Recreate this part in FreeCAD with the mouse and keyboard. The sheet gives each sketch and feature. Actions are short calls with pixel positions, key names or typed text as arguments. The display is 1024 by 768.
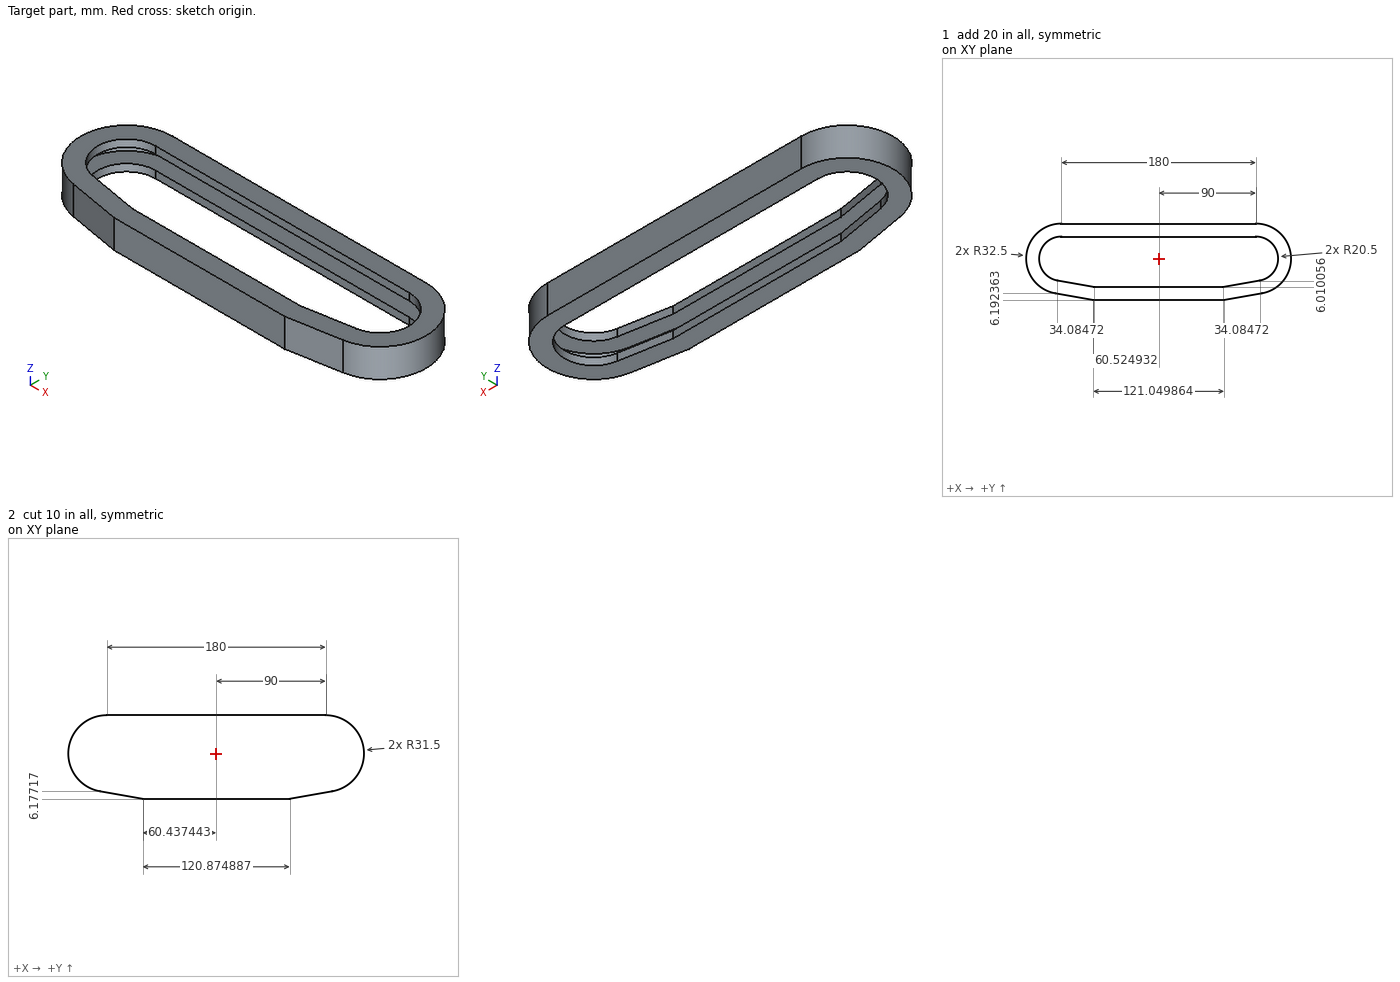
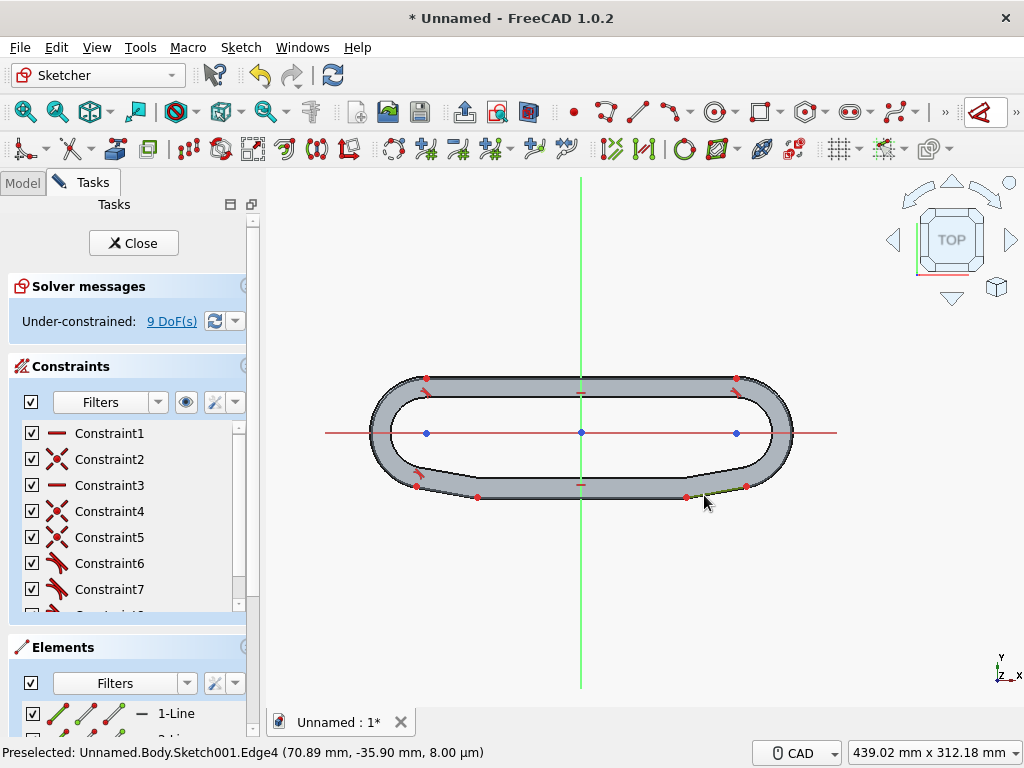
click(784, 460)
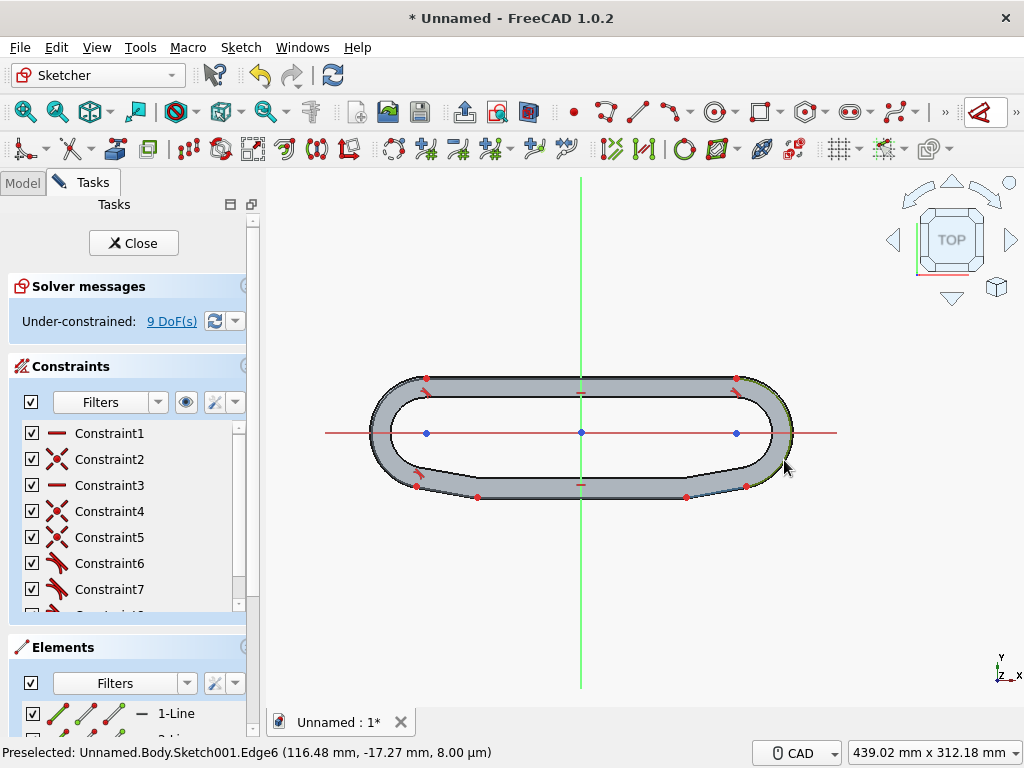
key(t)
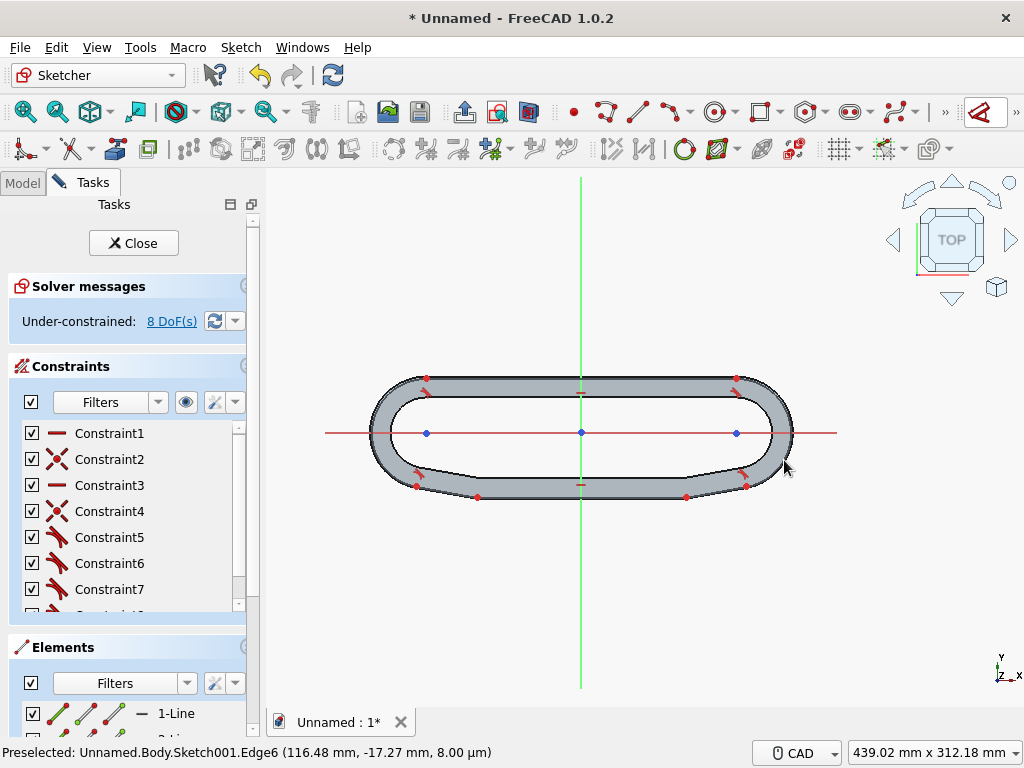
click(384, 399)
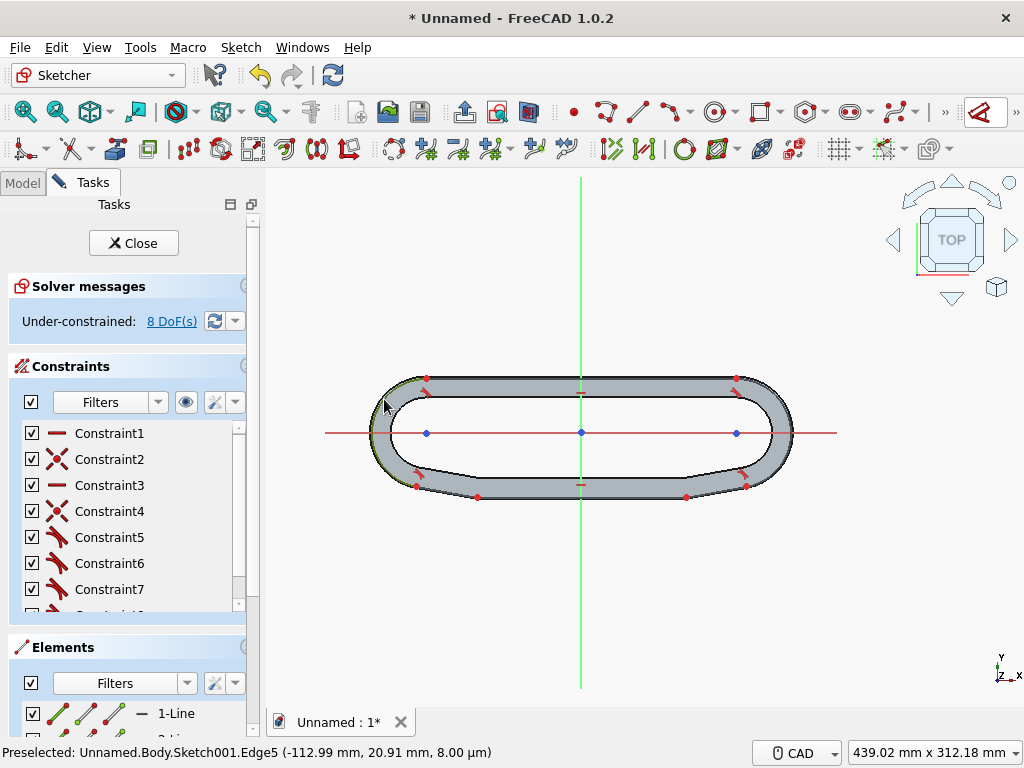
click(784, 460)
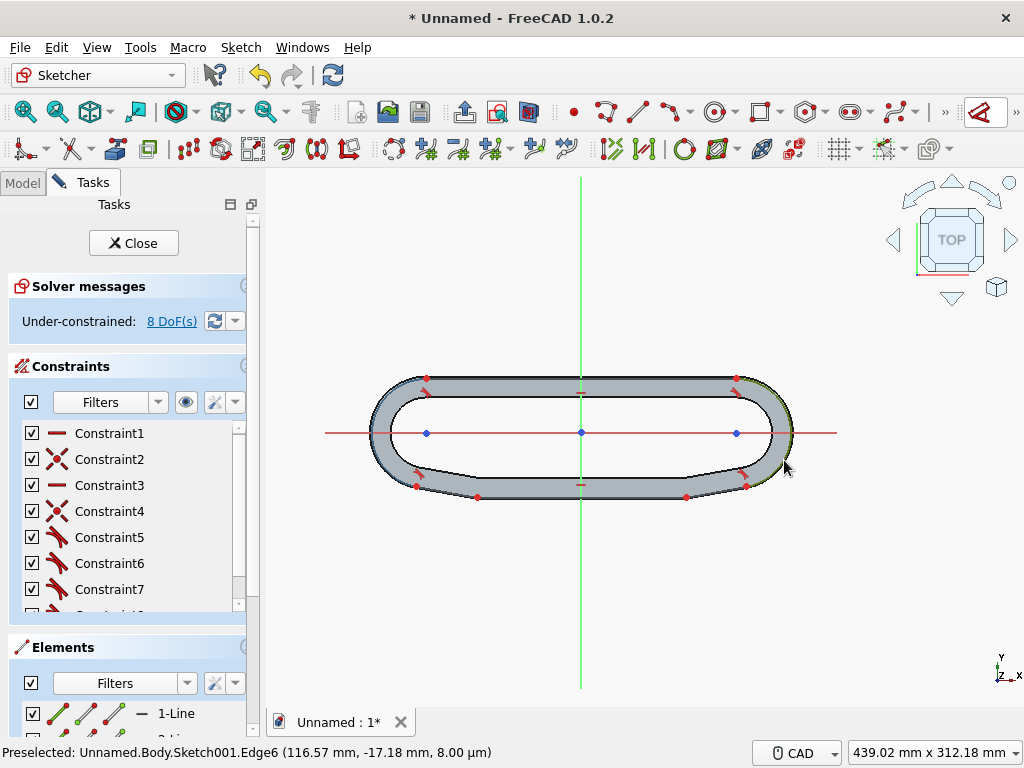
key(e)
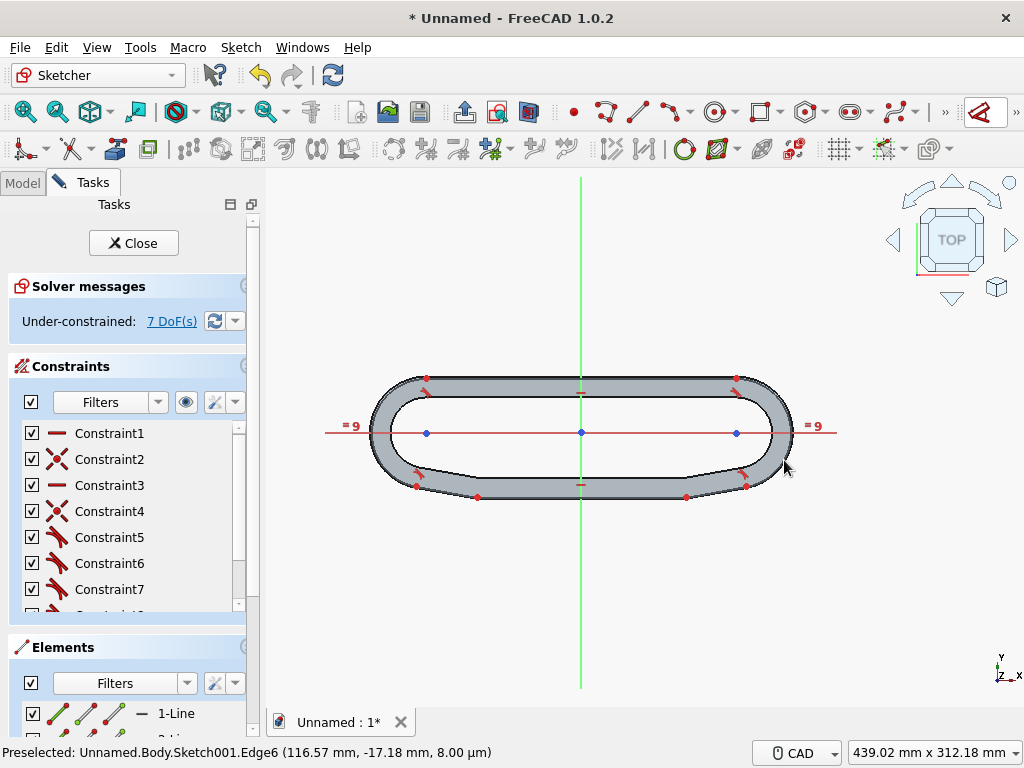
click(426, 433)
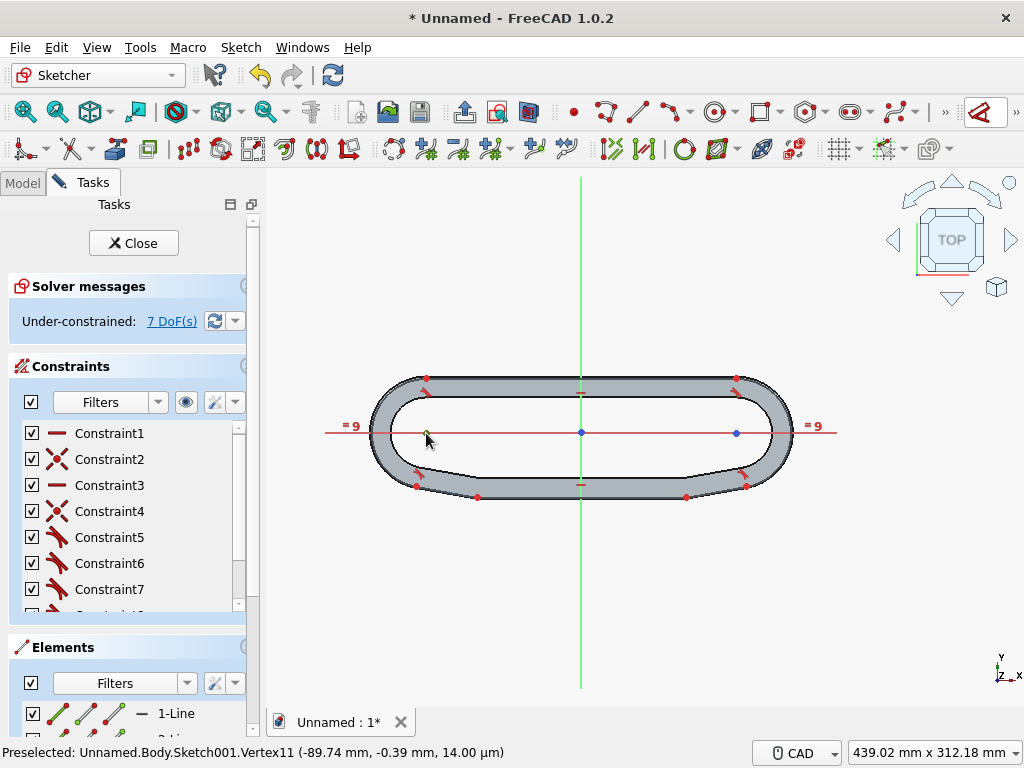
click(334, 433)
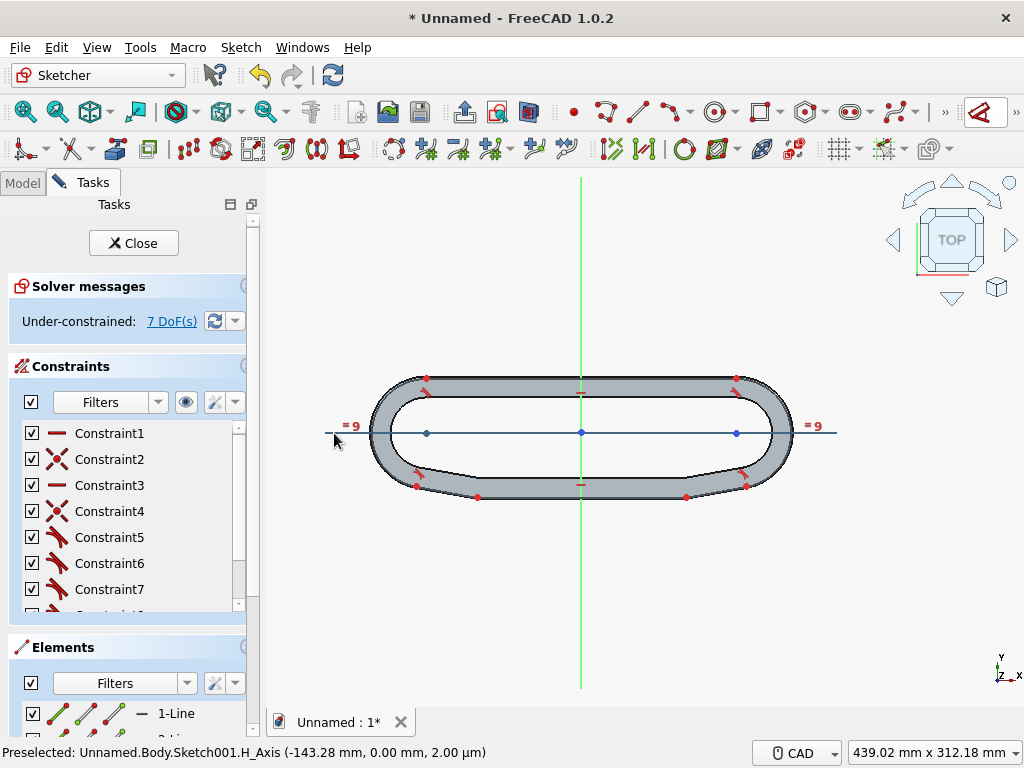
key(c)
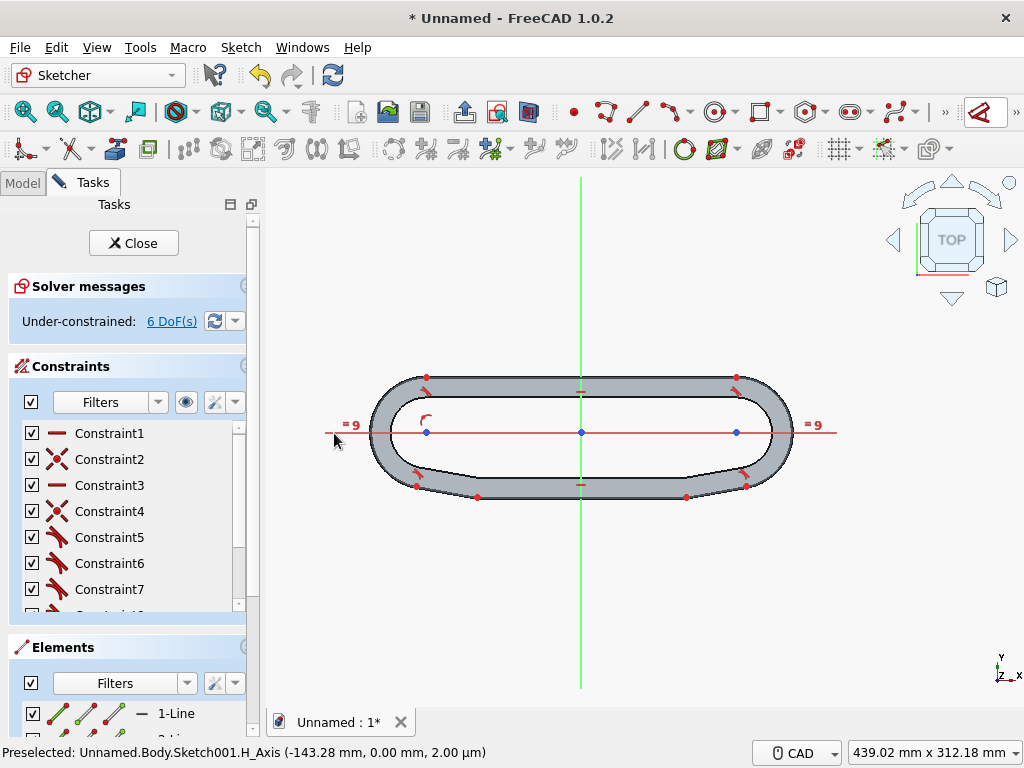
click(980, 112)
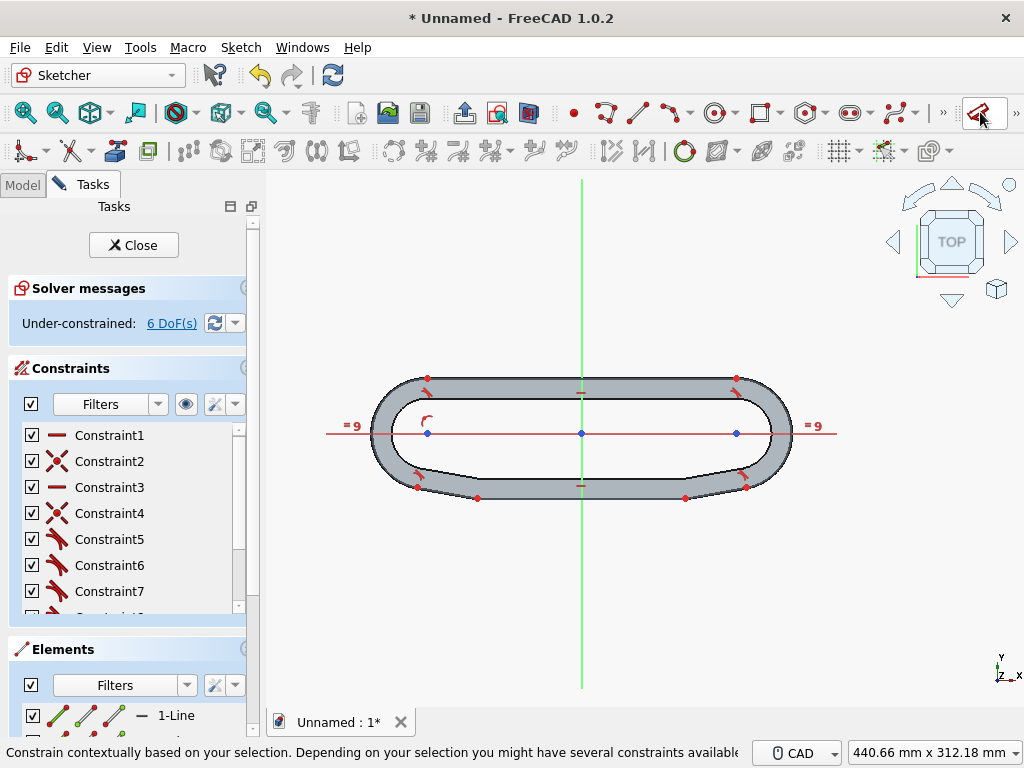
click(385, 399)
click(360, 379)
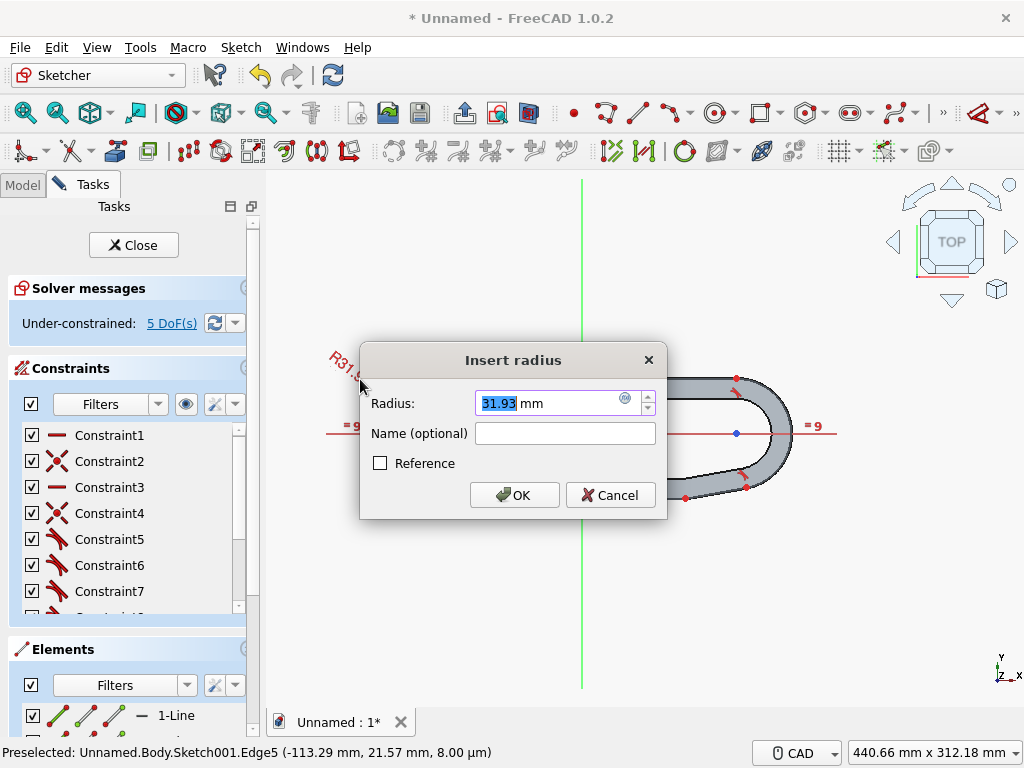
text(31.5)
key(Return)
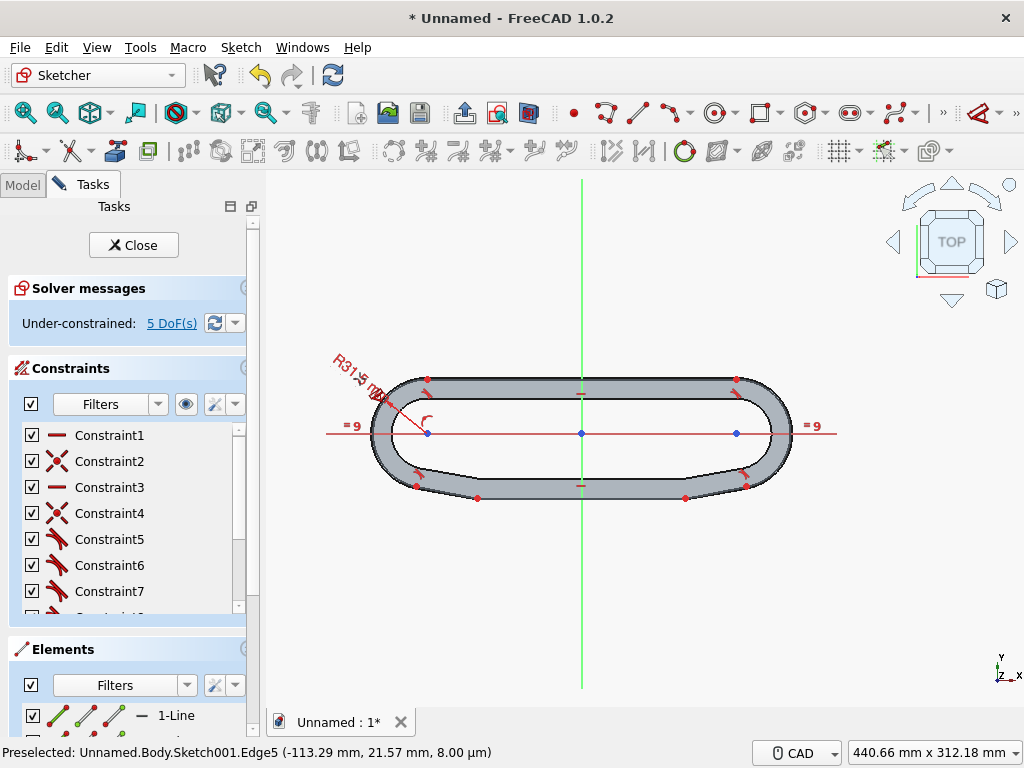
click(644, 380)
click(511, 346)